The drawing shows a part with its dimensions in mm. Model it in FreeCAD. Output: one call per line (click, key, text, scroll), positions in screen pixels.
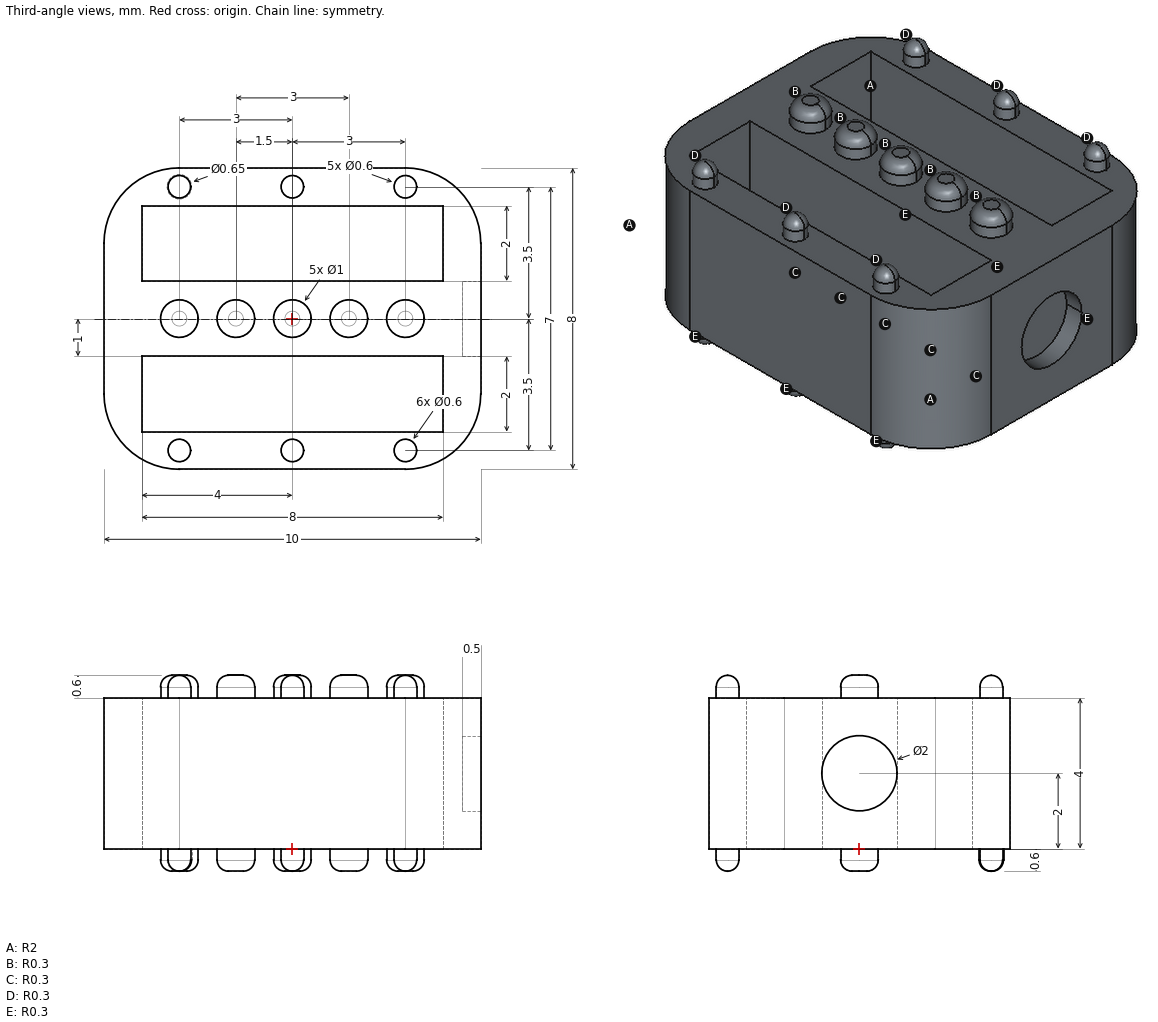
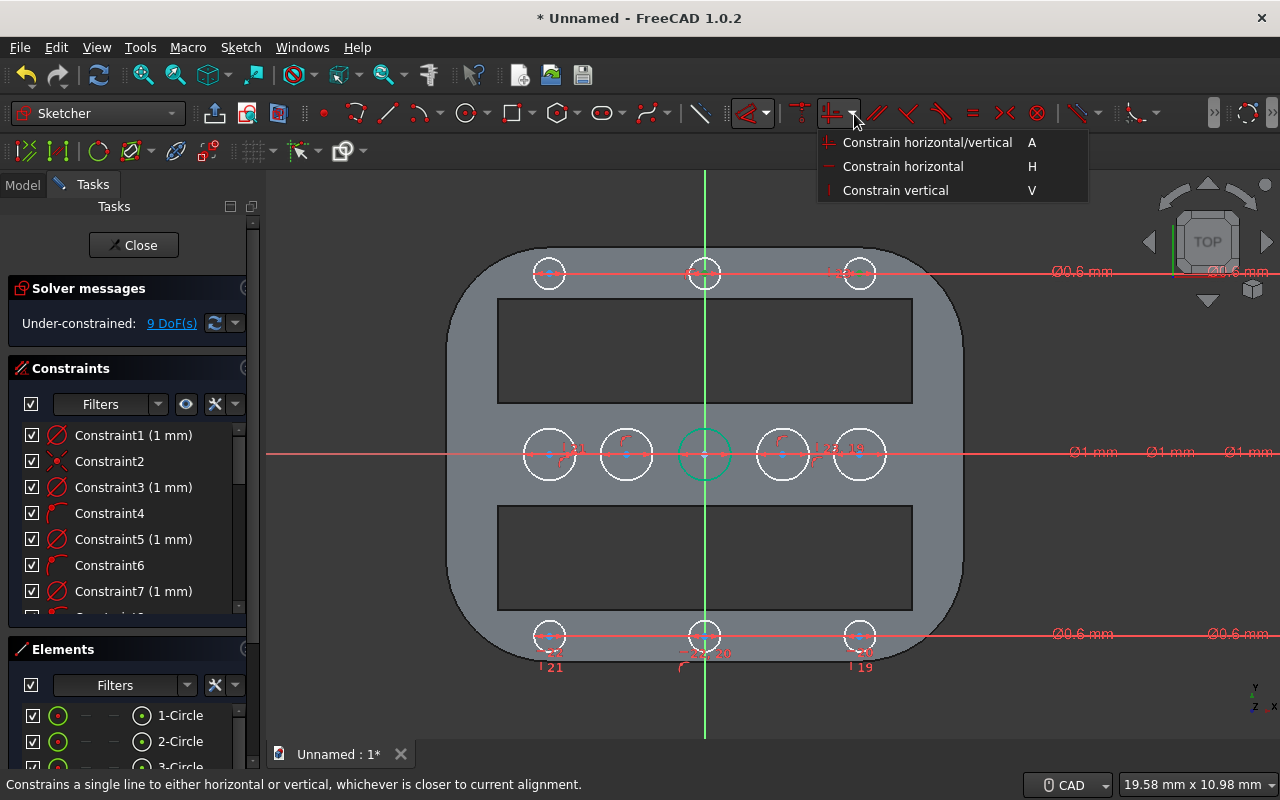
click(953, 166)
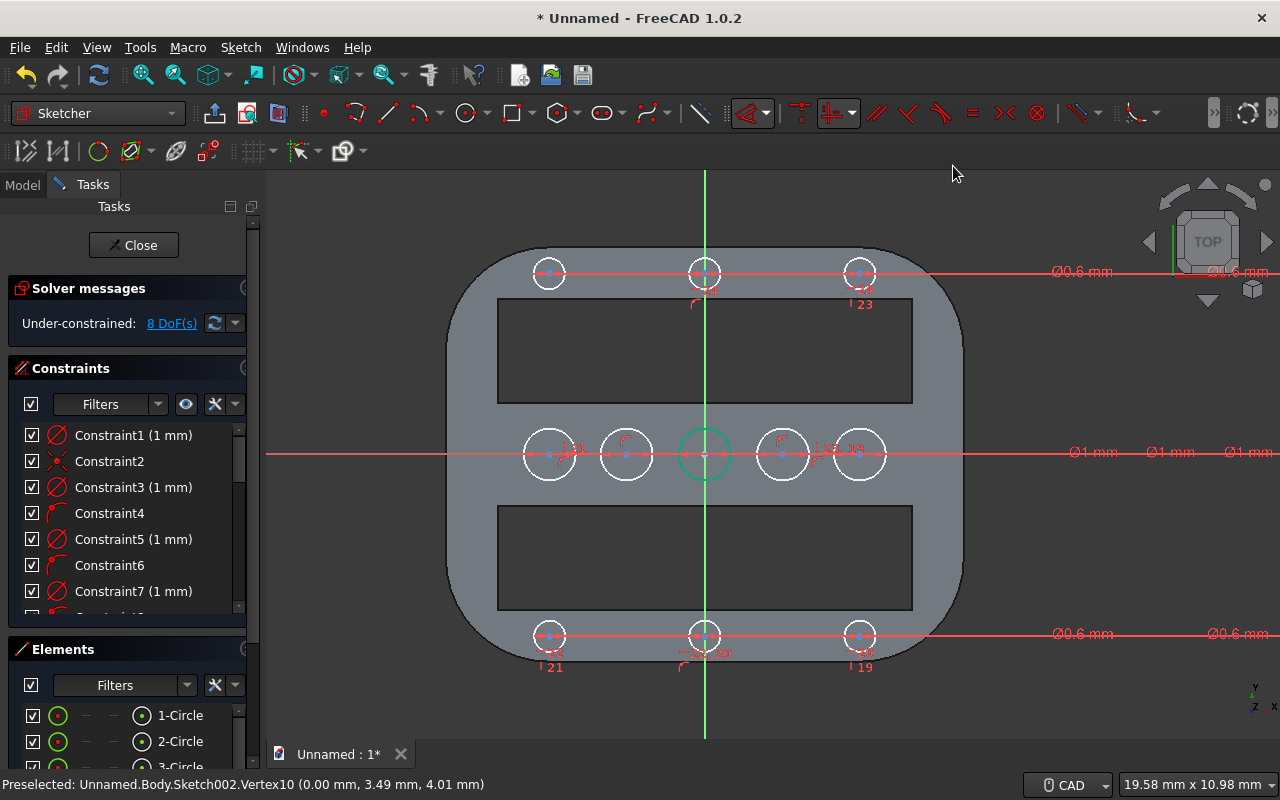
click(550, 454)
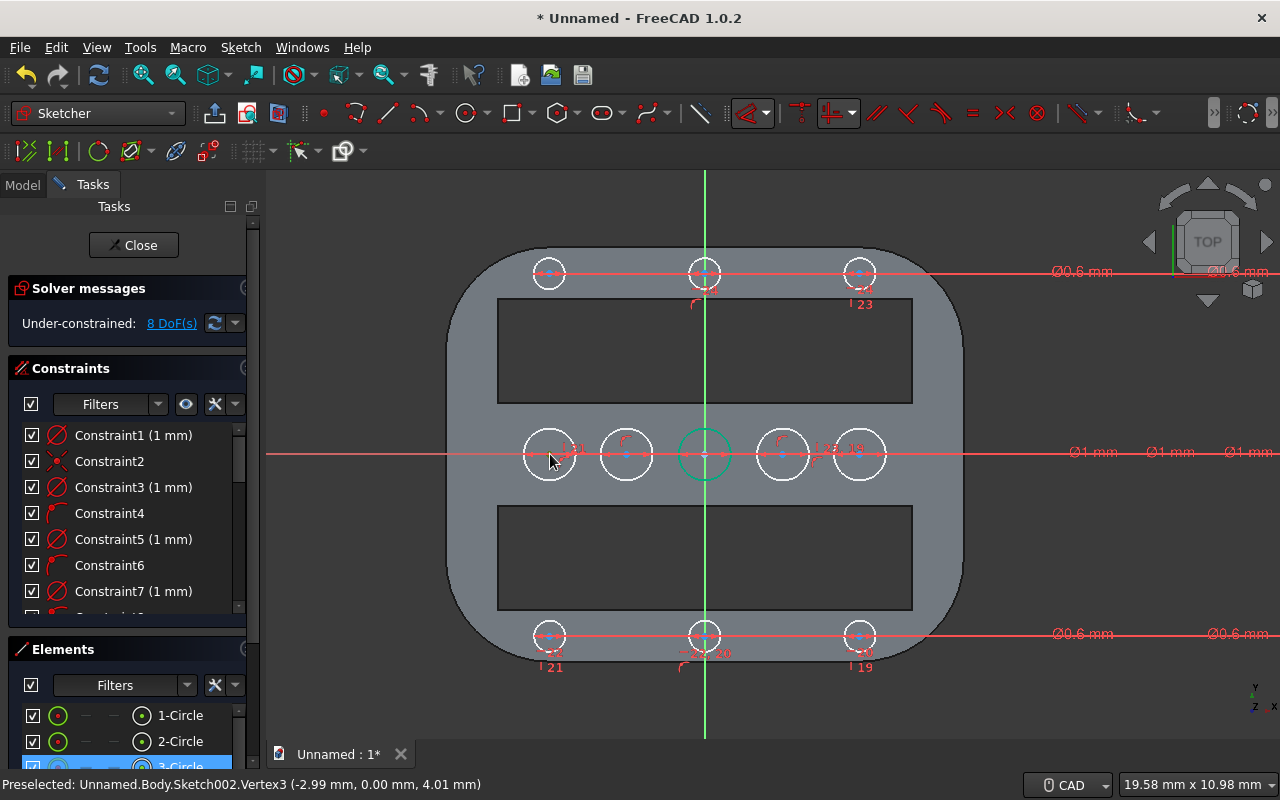
click(549, 274)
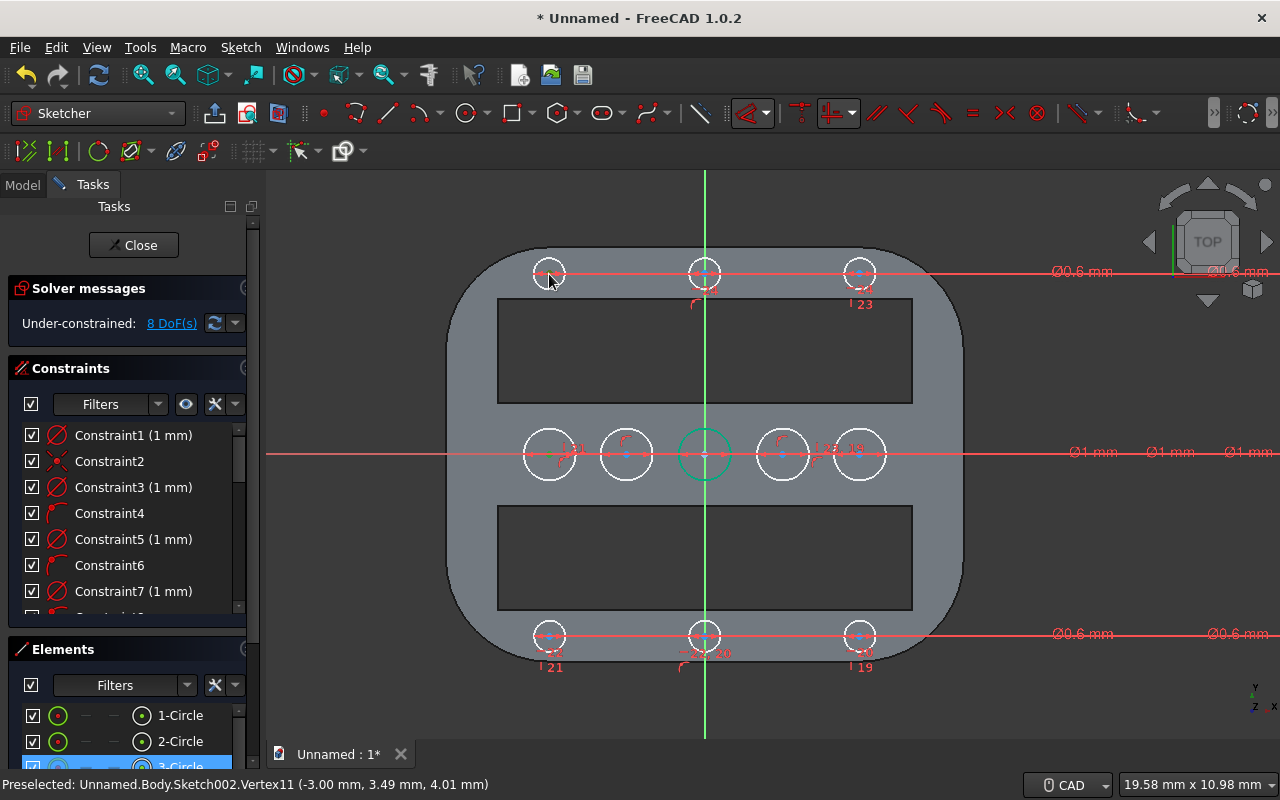
key(v)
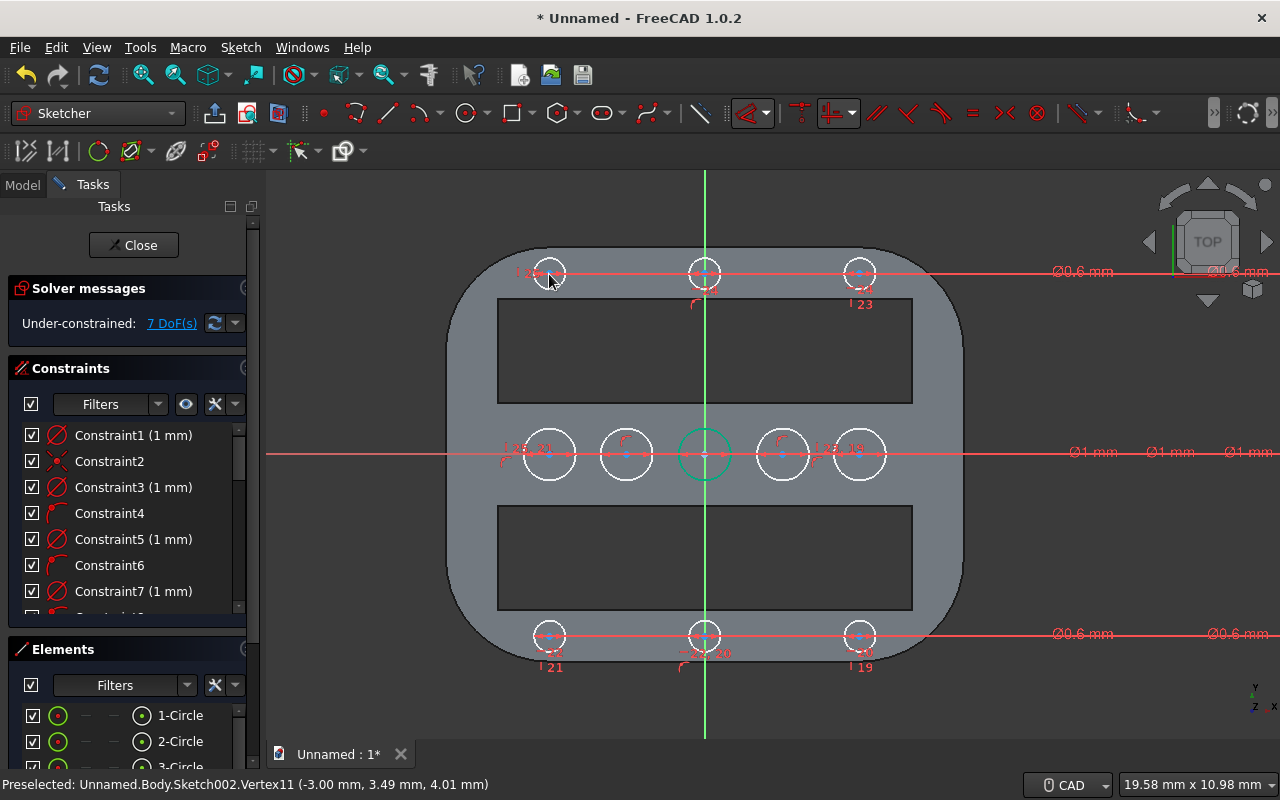
click(705, 274)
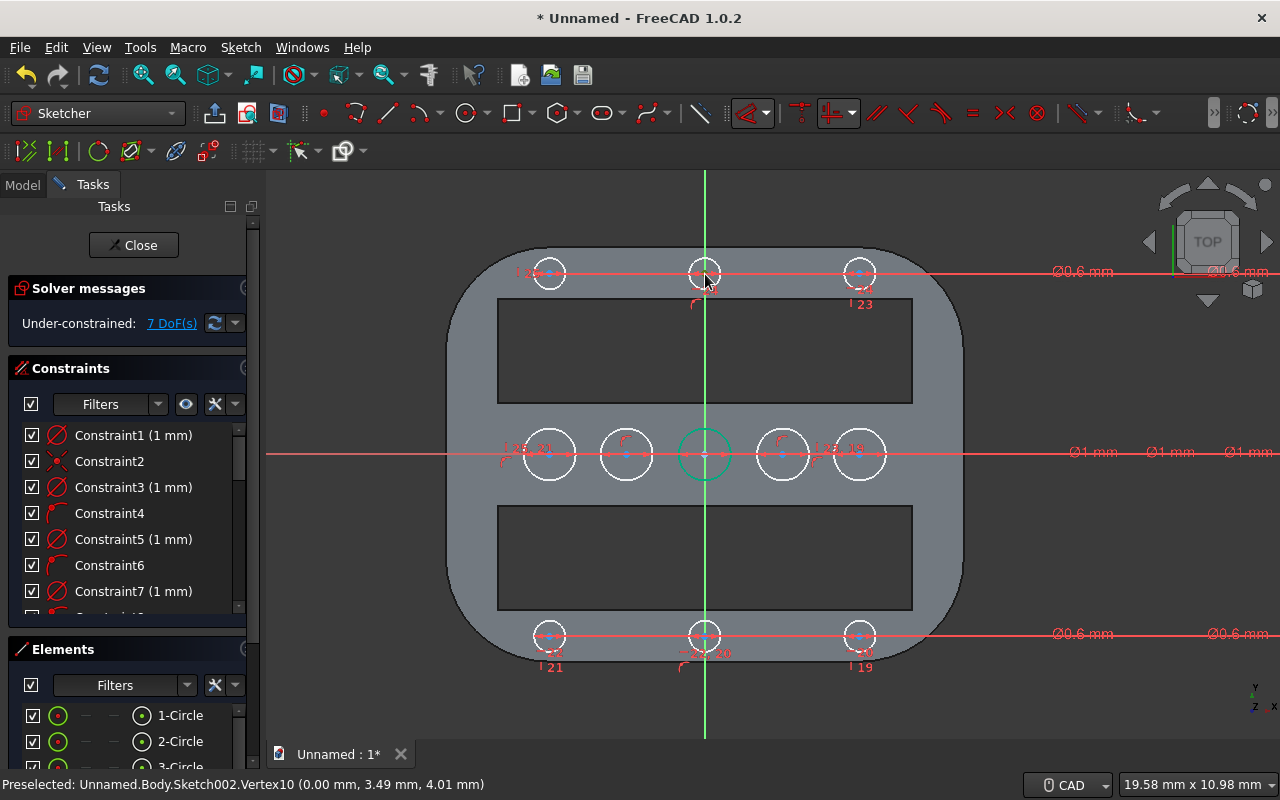
click(550, 274)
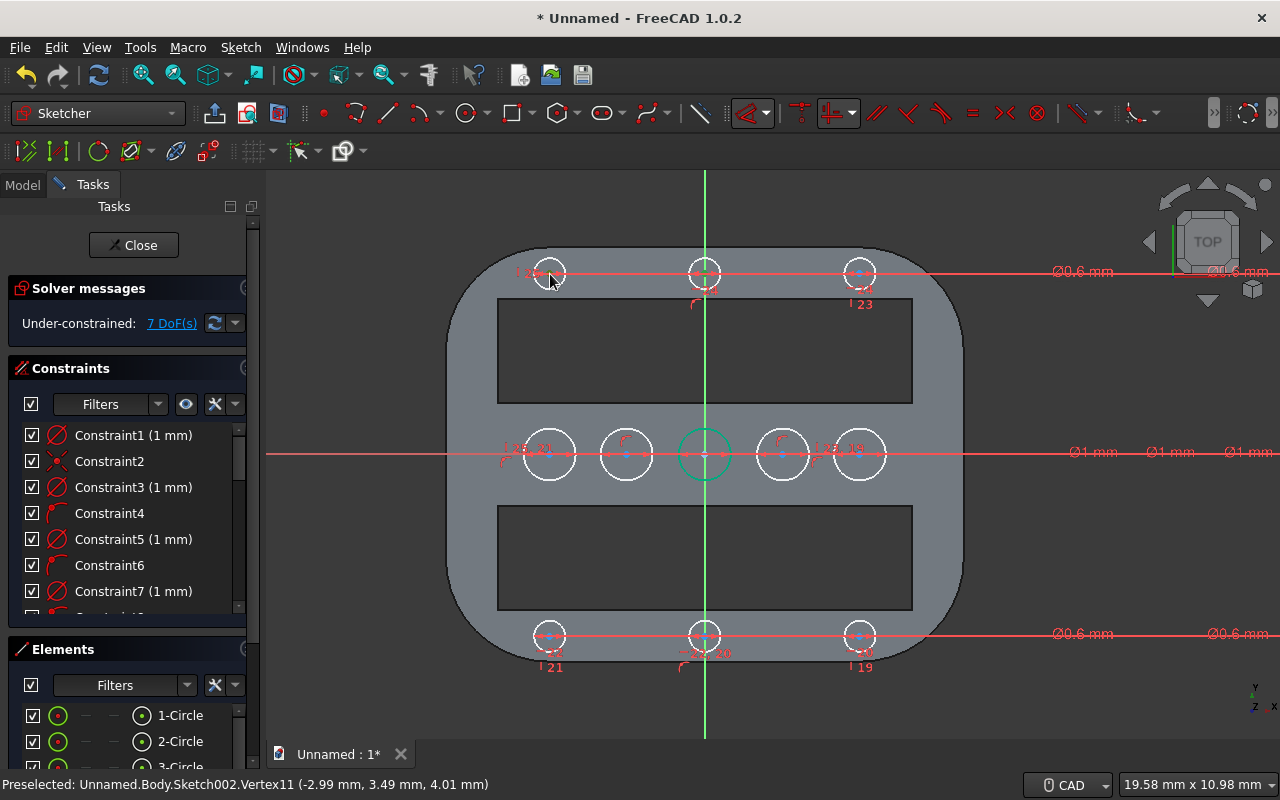
click(854, 114)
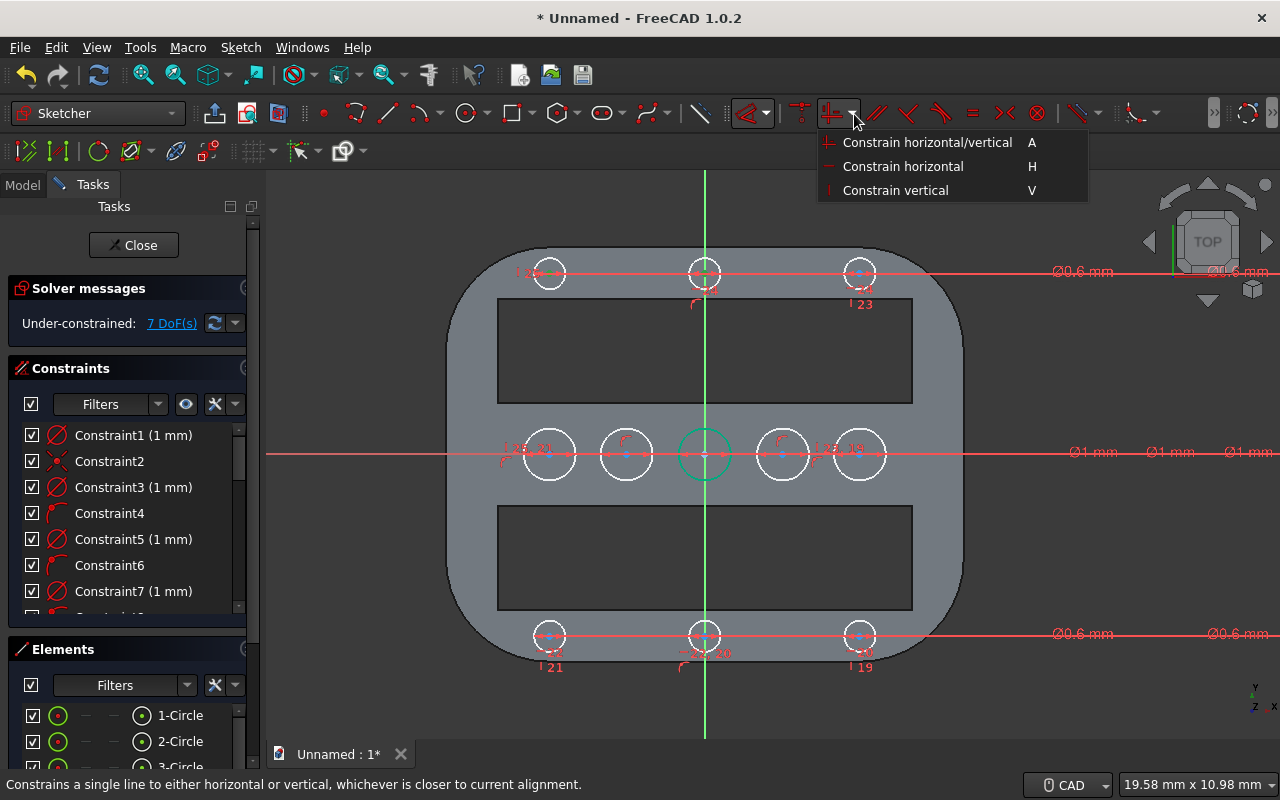
click(953, 166)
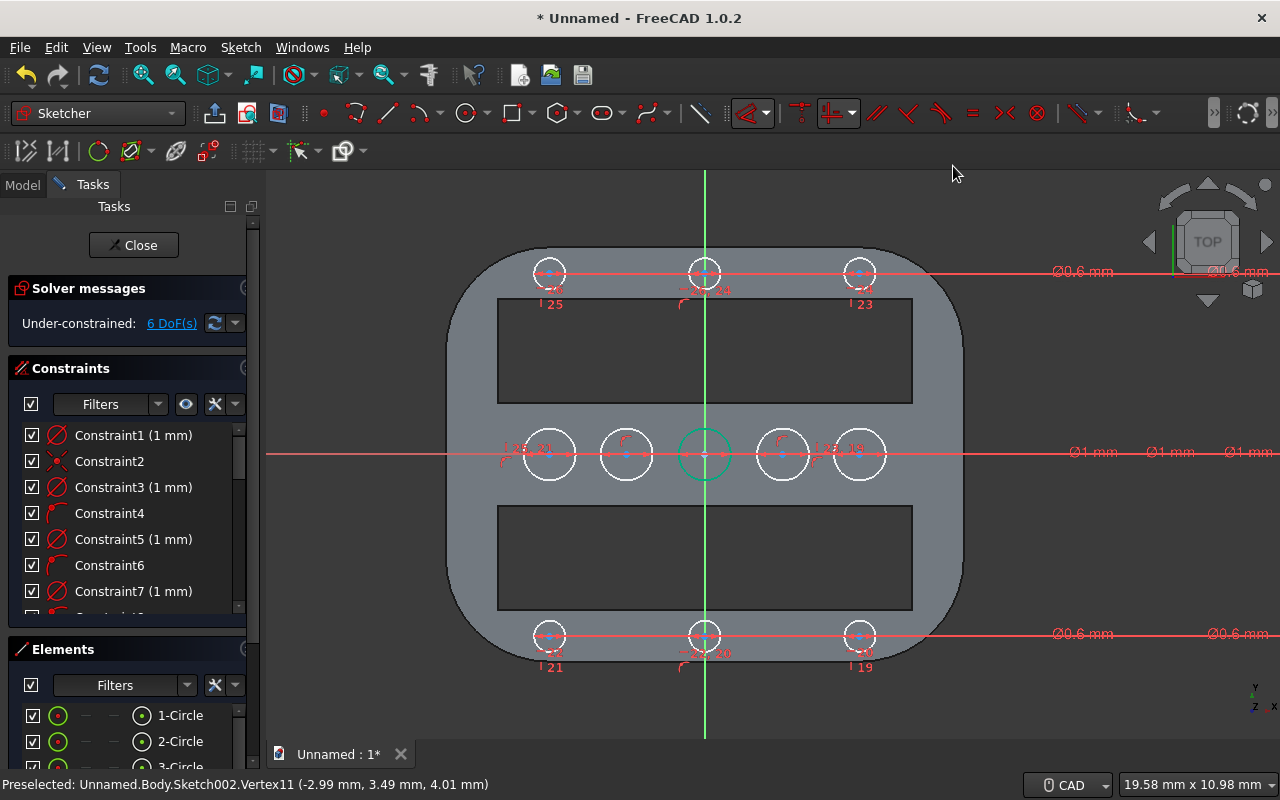
click(550, 454)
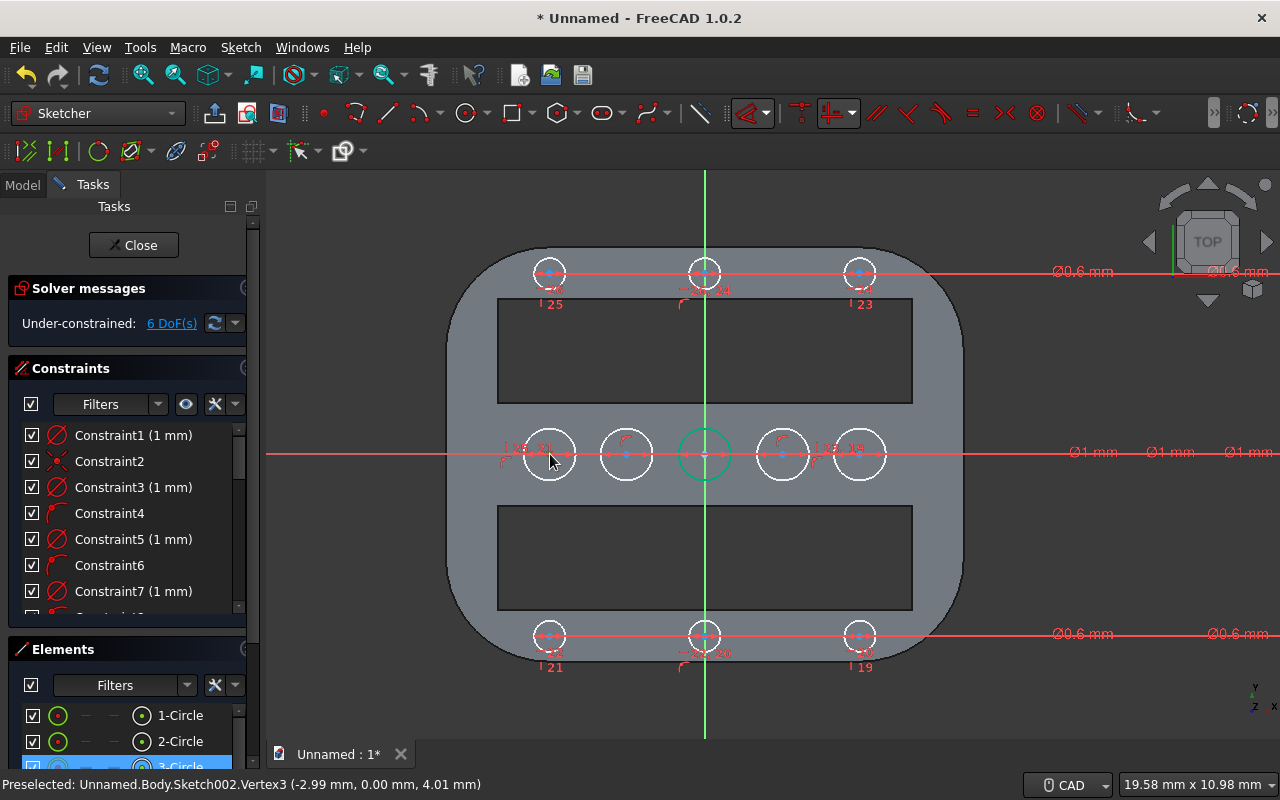
key(l)